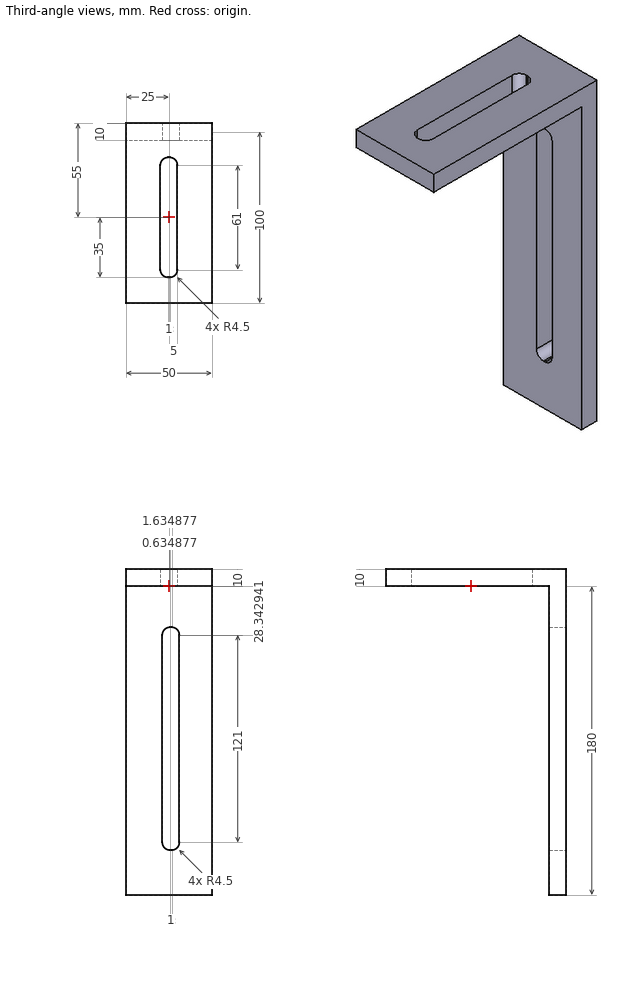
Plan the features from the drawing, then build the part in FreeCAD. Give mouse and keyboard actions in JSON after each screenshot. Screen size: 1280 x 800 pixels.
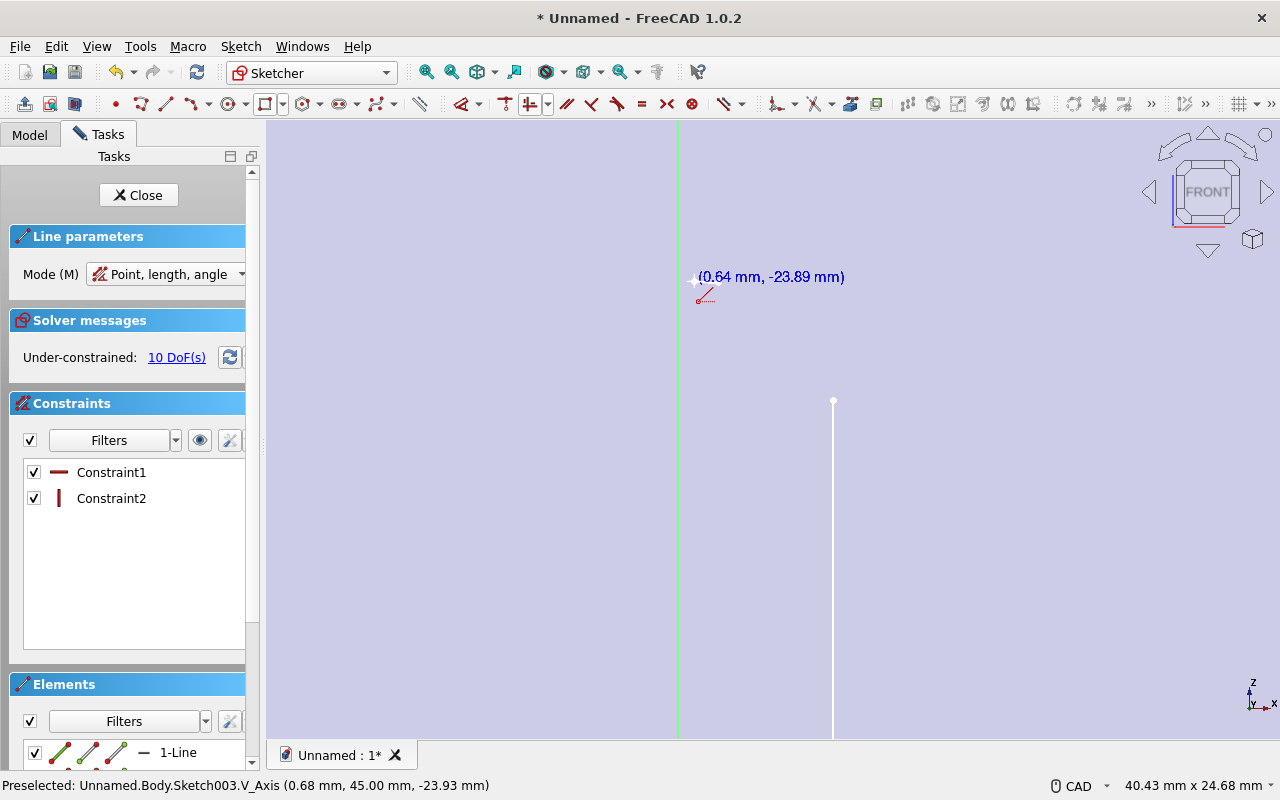
{"action": "scroll", "coordinate": [704, 282], "scroll_direction": "down", "scroll_amount": 11}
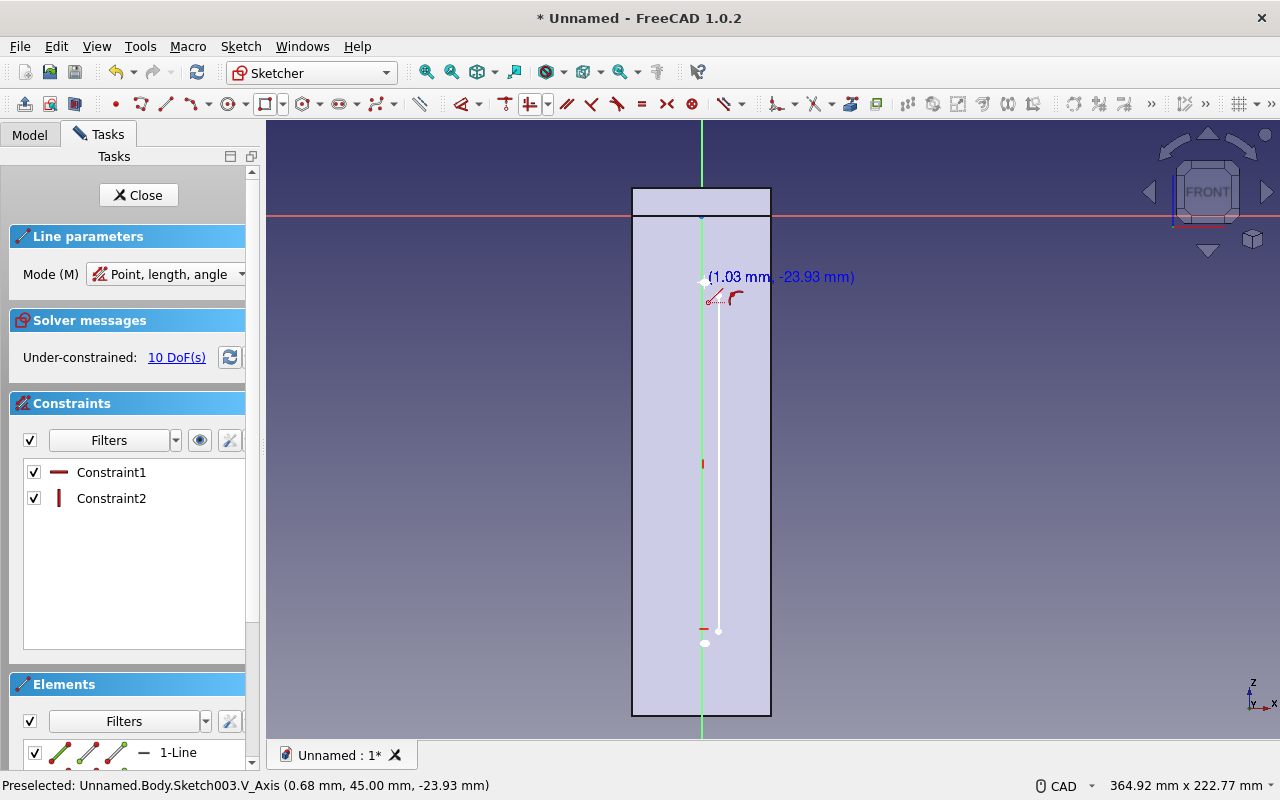
{"action": "scroll", "coordinate": [691, 295], "scroll_direction": "up", "scroll_amount": 2}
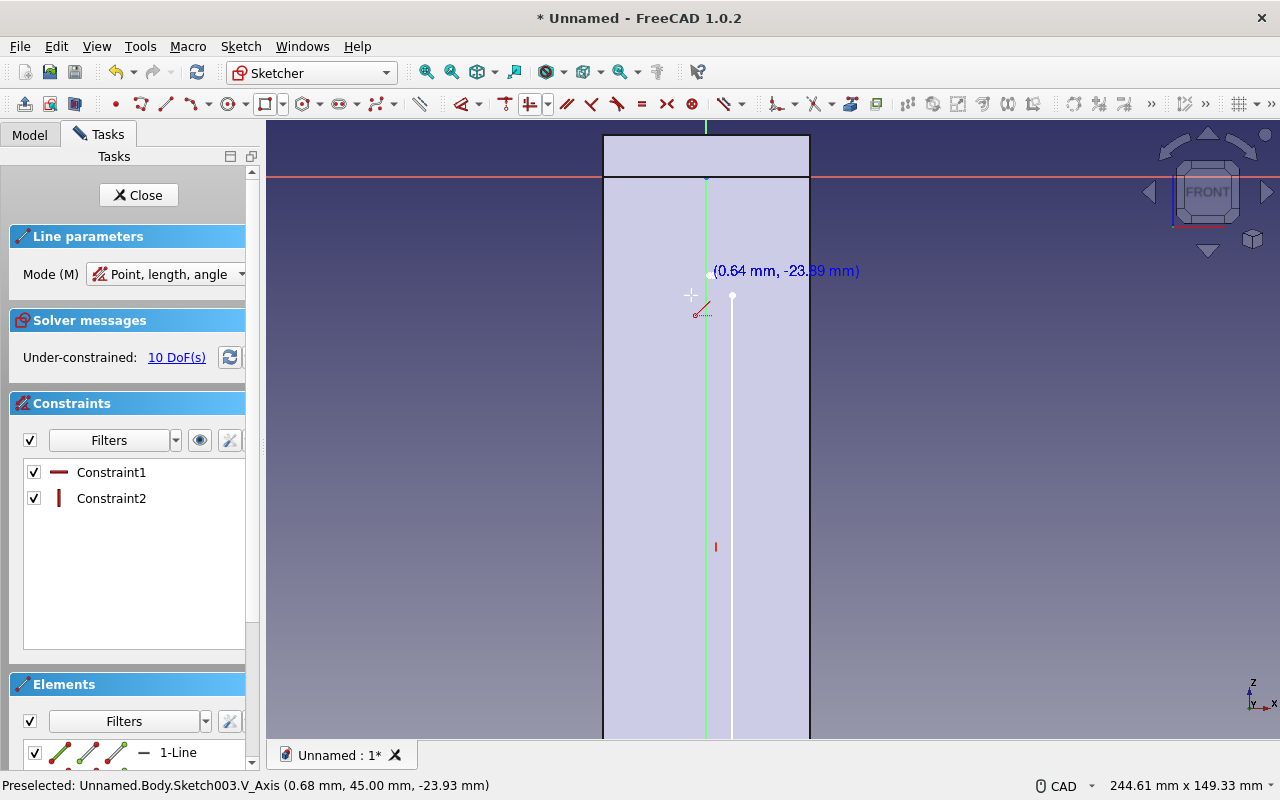
{"action": "left_click", "coordinate": [690, 294]}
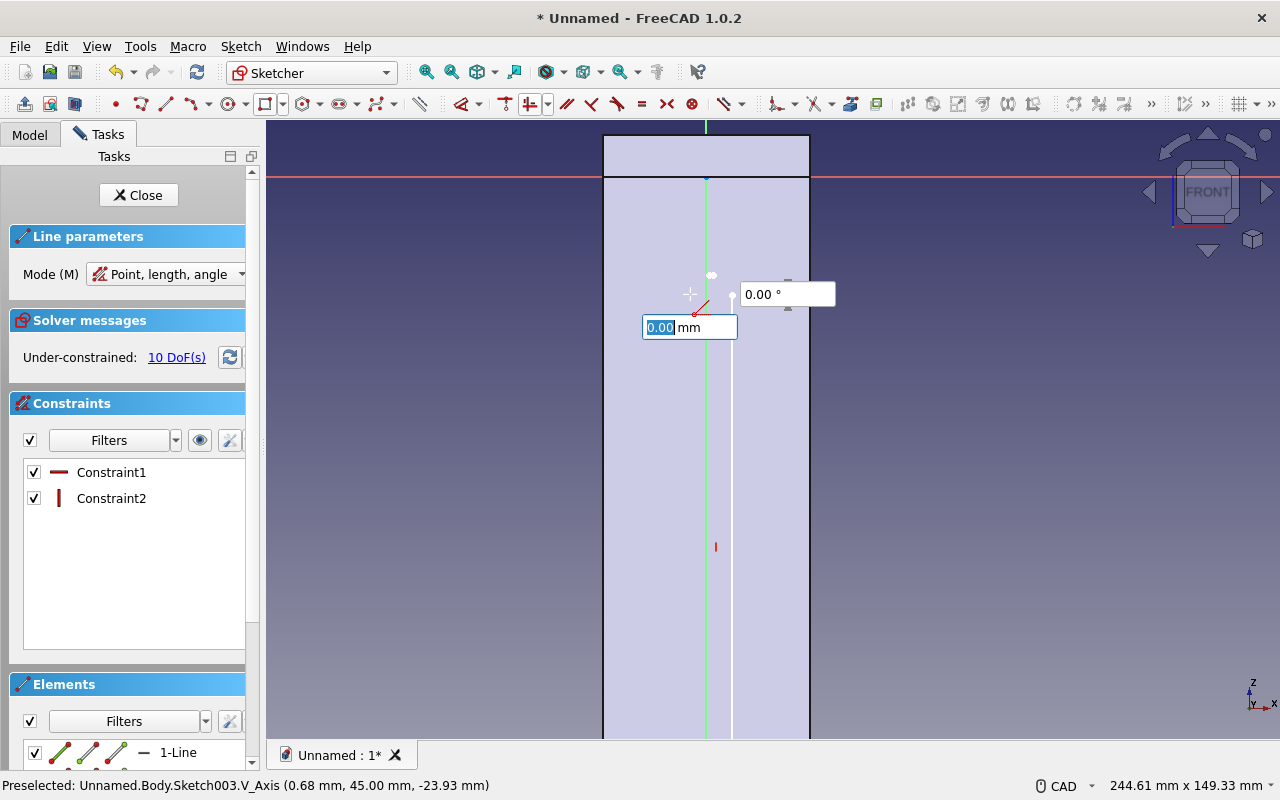
{"action": "scroll", "coordinate": [691, 295], "scroll_direction": "down", "scroll_amount": 2}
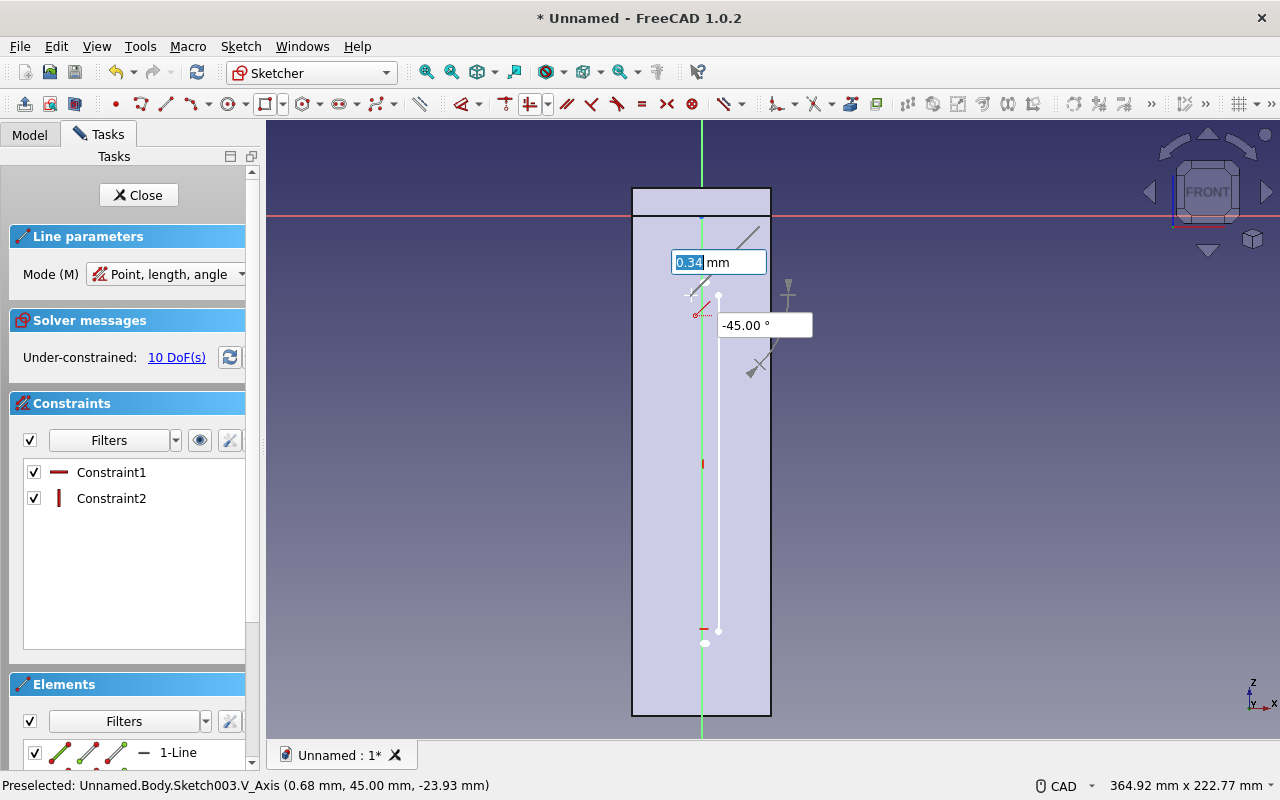
{"action": "scroll", "coordinate": [691, 631], "scroll_direction": "up", "scroll_amount": 2}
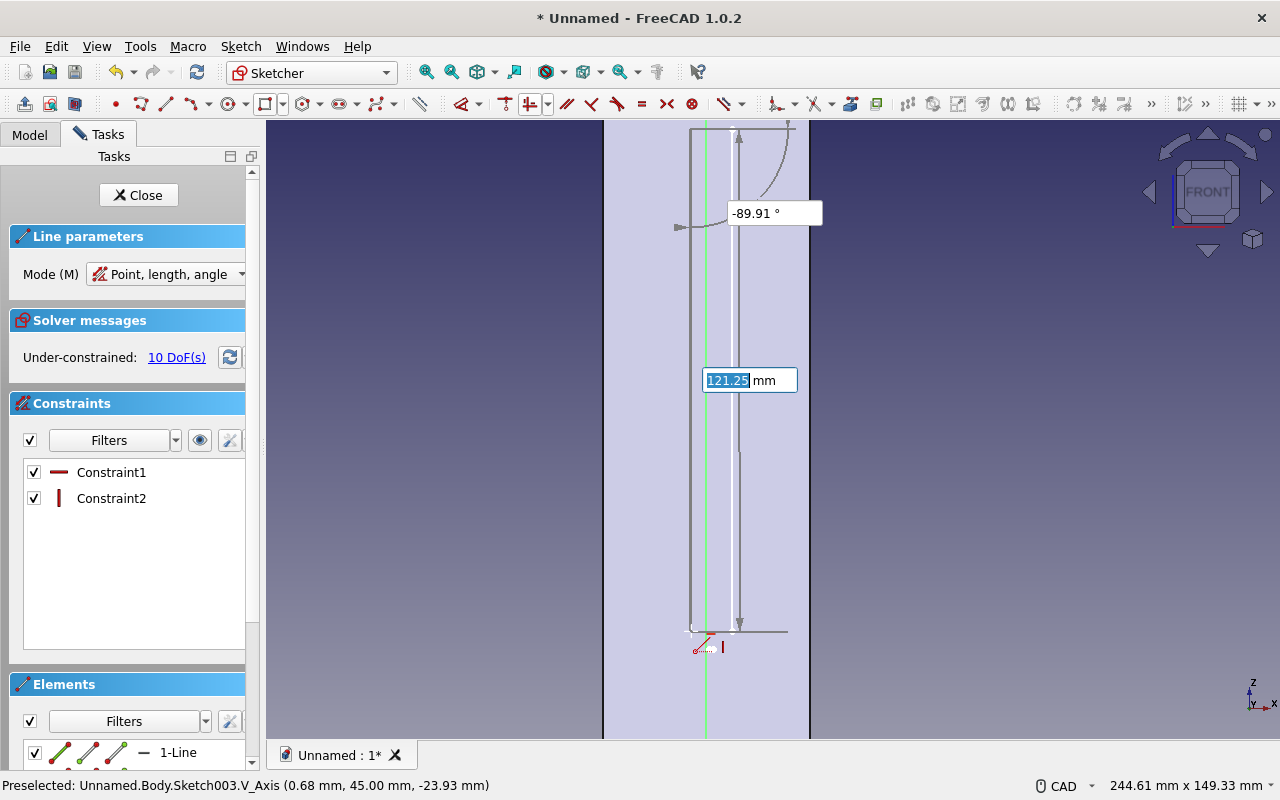
{"action": "left_click", "coordinate": [690, 630]}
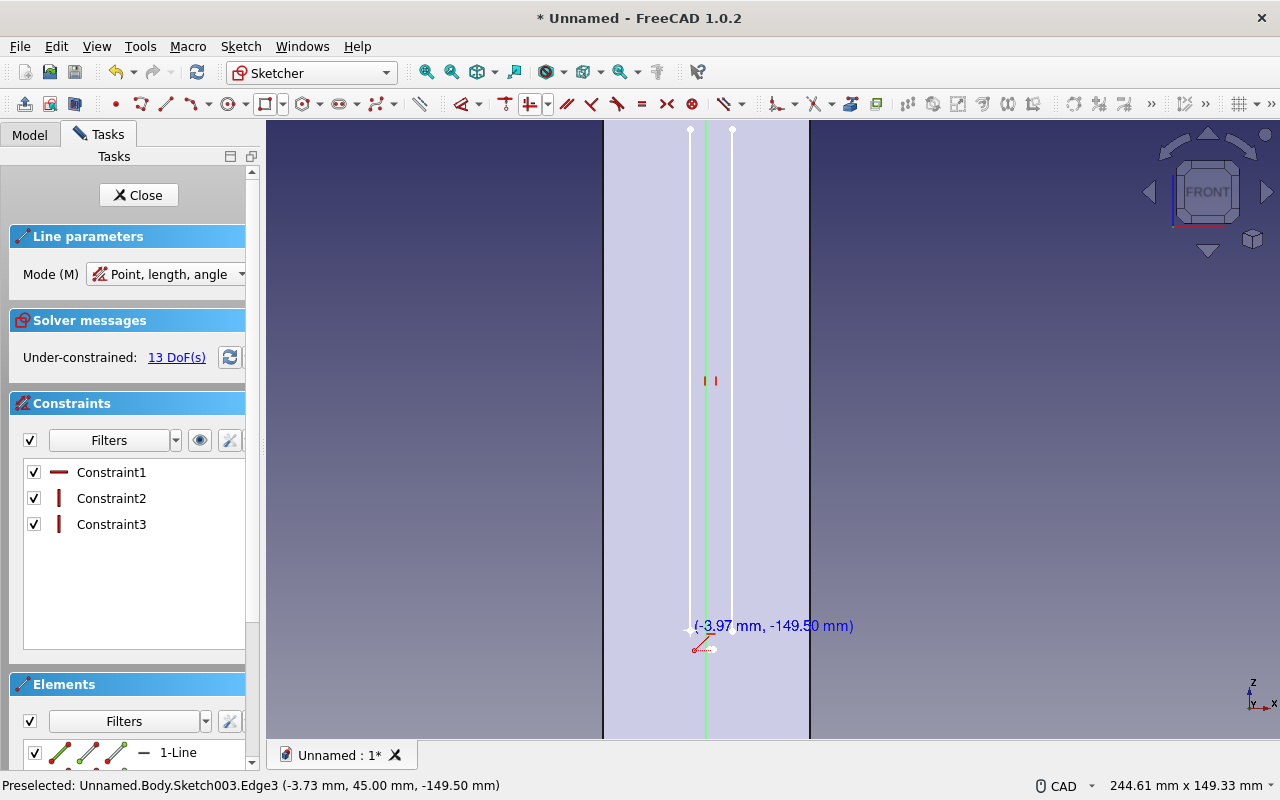
{"action": "left_click", "coordinate": [190, 104]}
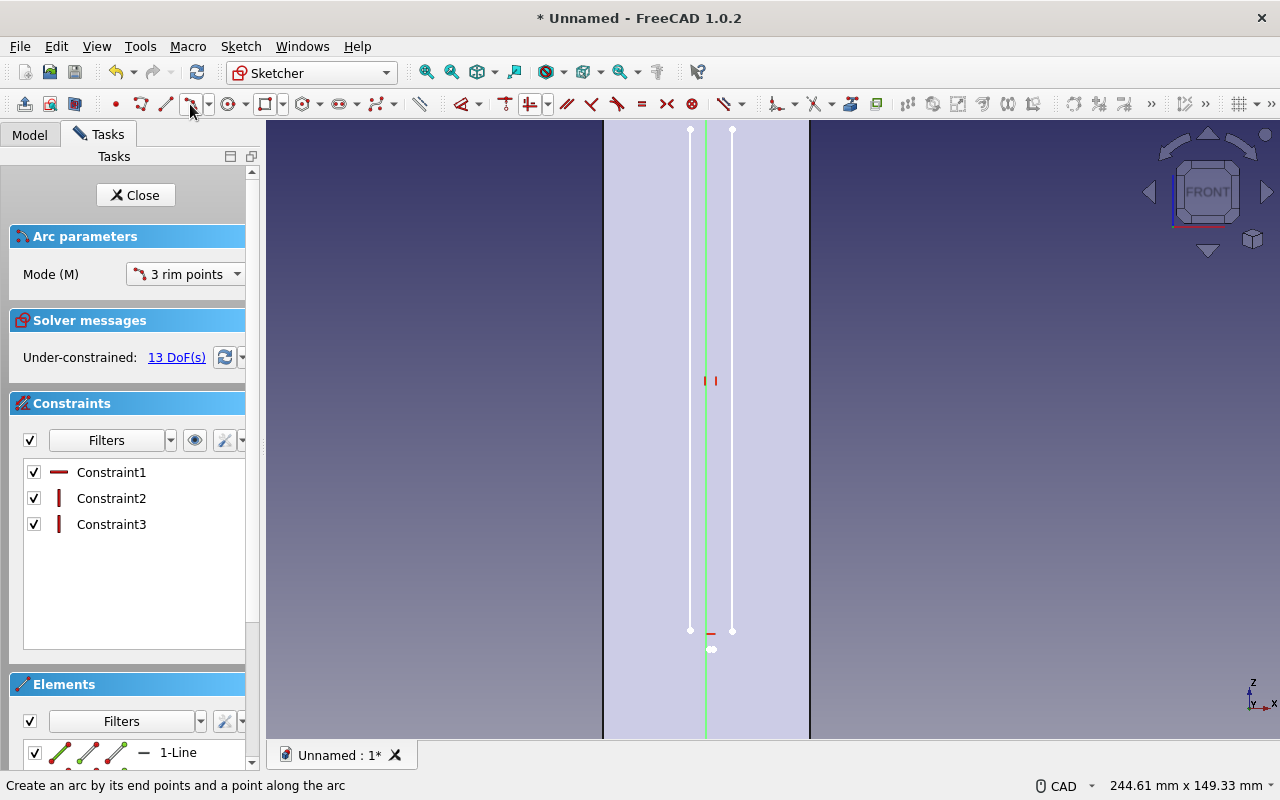
{"action": "scroll", "coordinate": [713, 649], "scroll_direction": "up", "scroll_amount": 11}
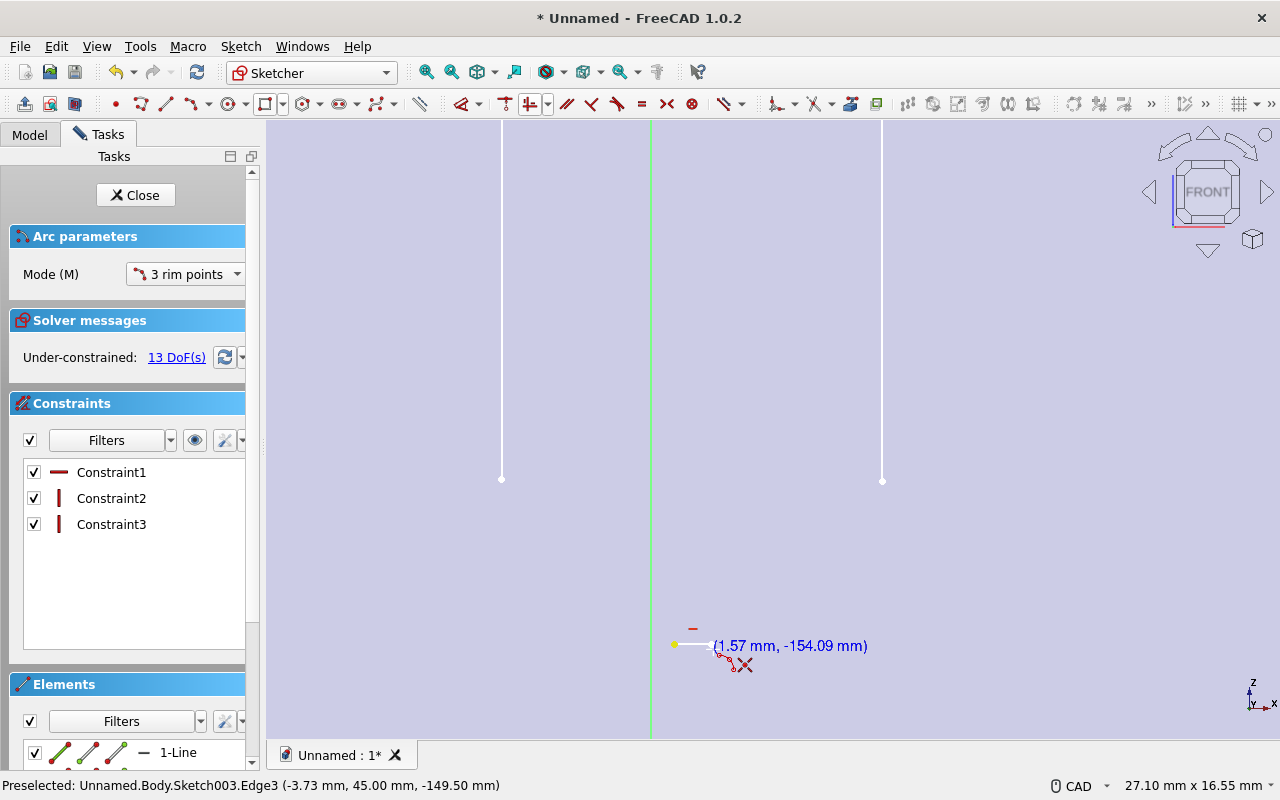
{"action": "left_click", "coordinate": [712, 644]}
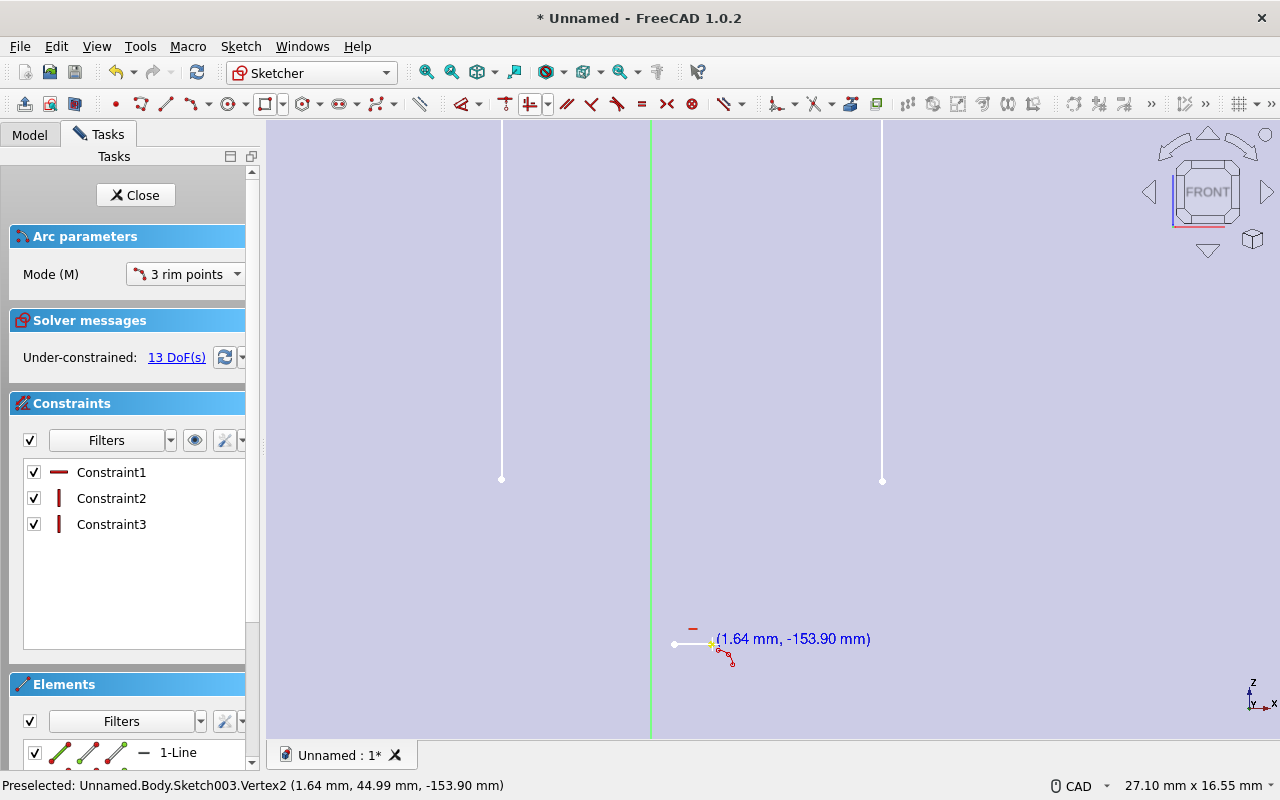
{"action": "scroll", "coordinate": [705, 643], "scroll_direction": "down", "scroll_amount": 13}